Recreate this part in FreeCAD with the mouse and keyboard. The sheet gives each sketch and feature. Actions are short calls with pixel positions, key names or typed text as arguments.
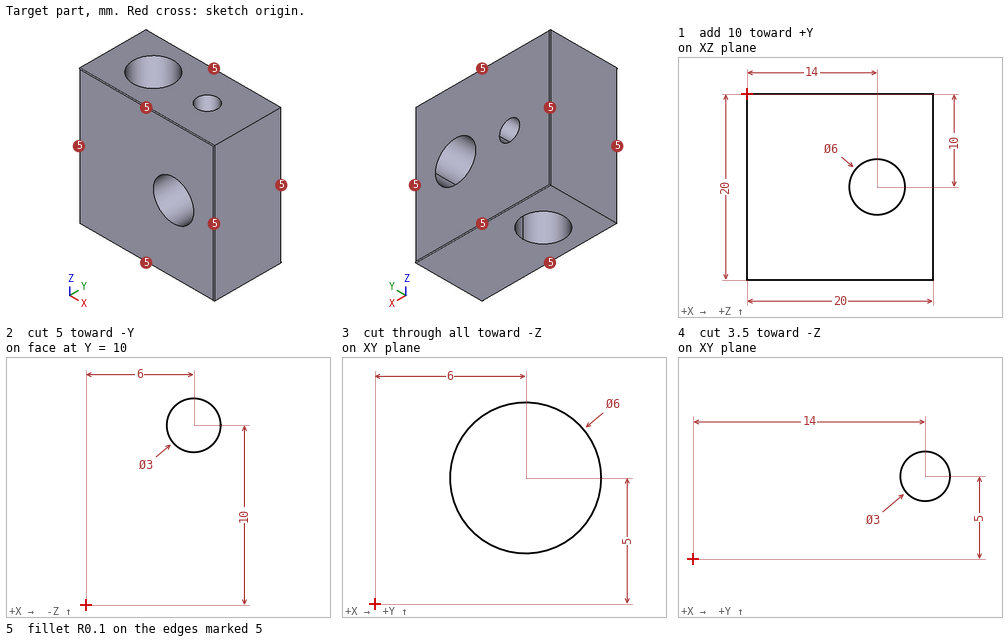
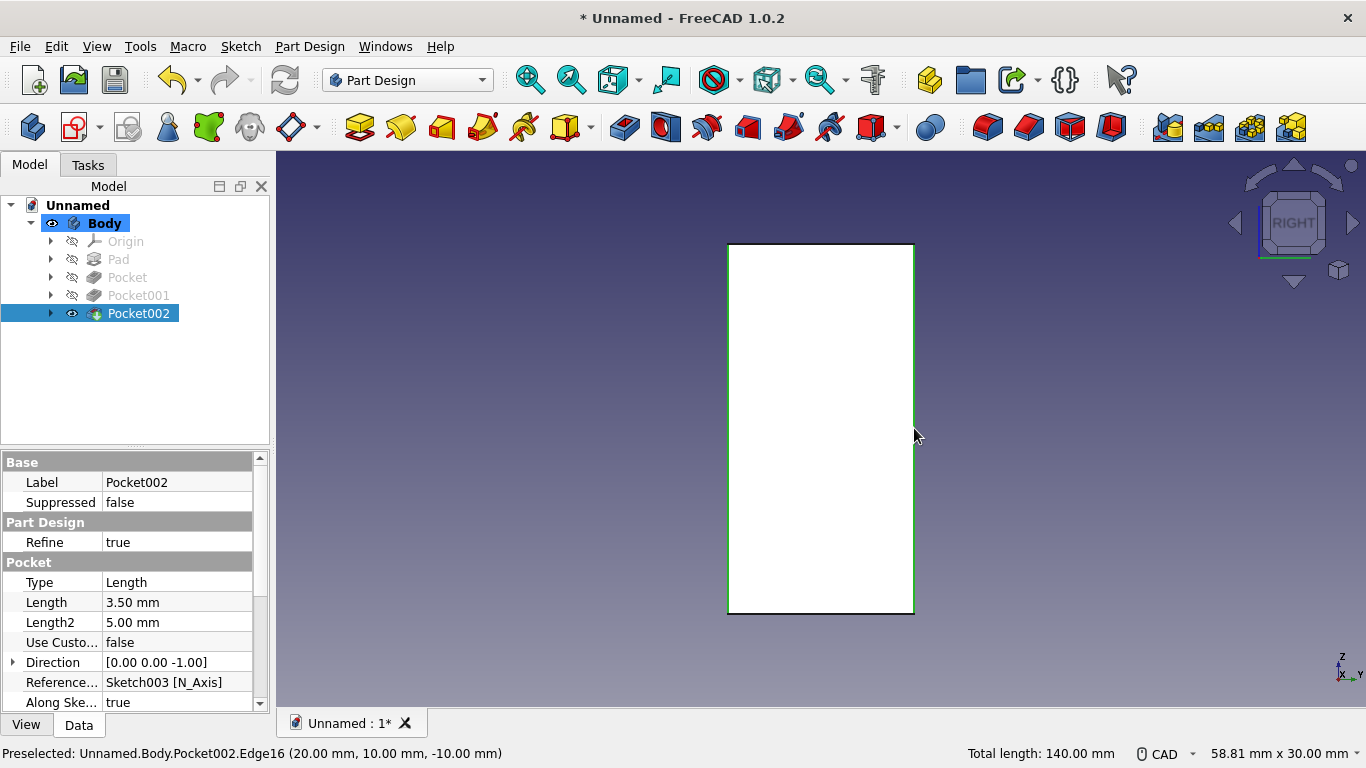
key(5)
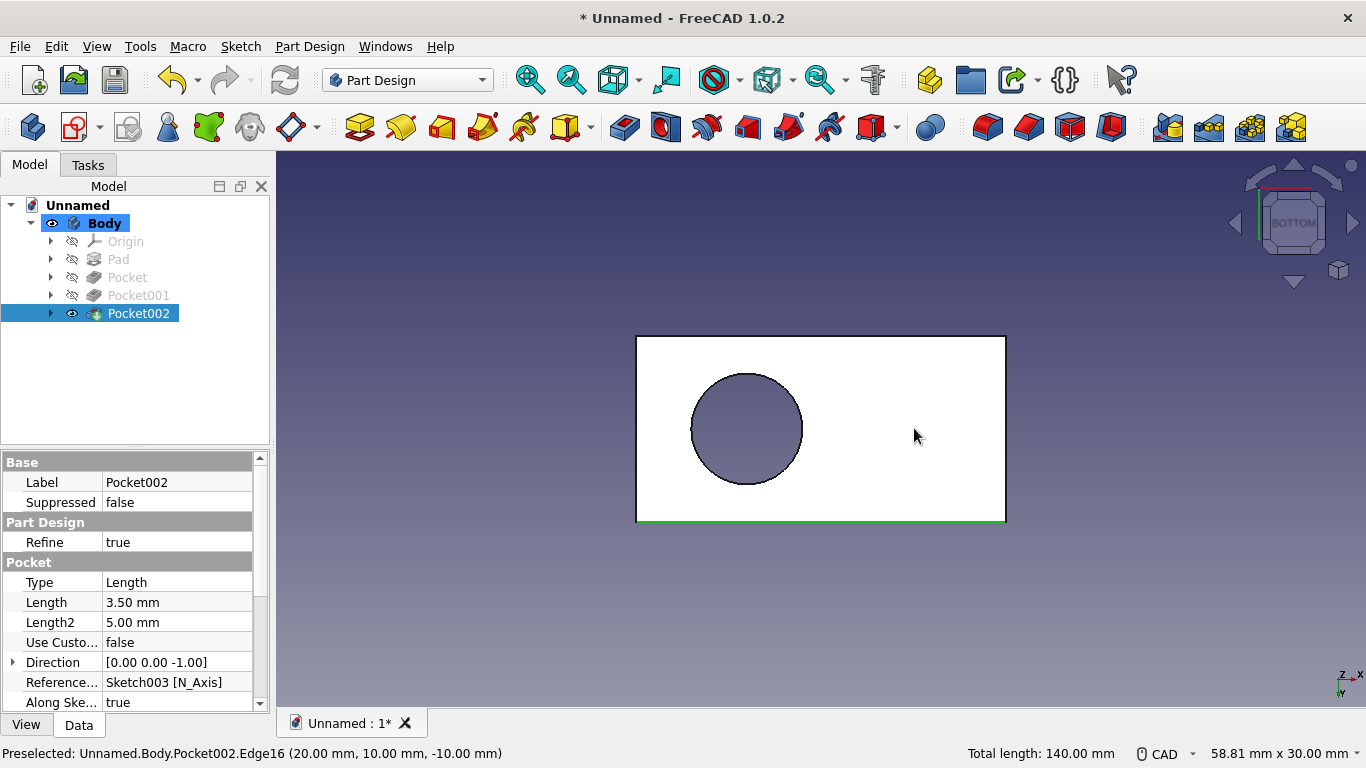
key(v)
key(f)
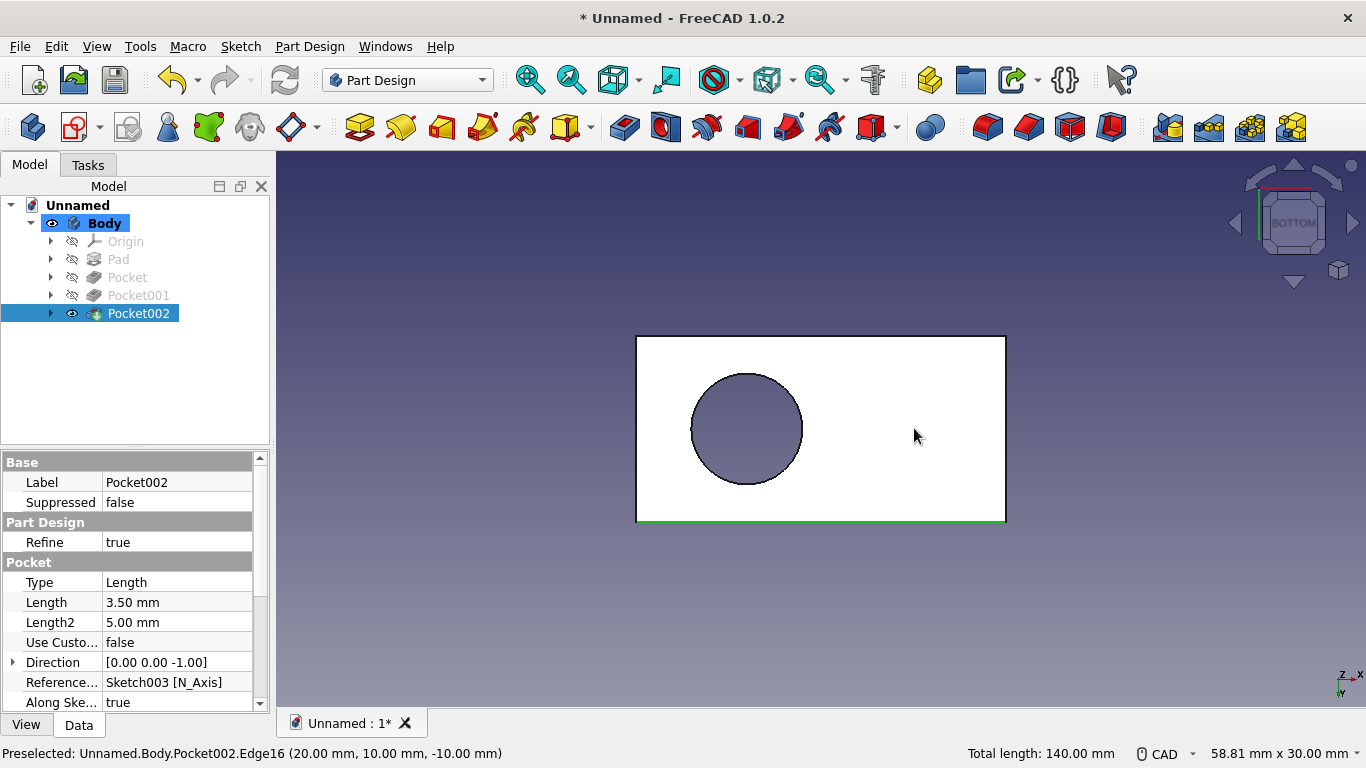
click(821, 335, ctrl)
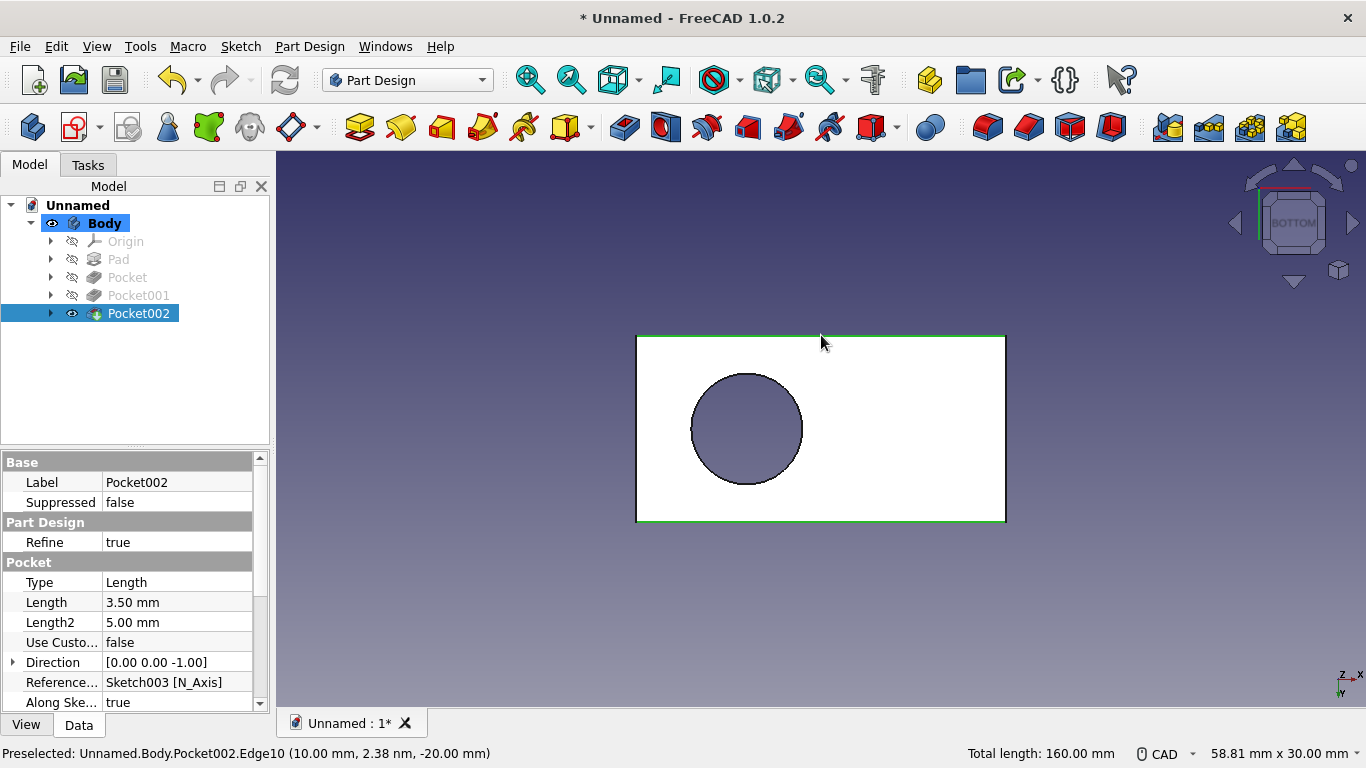
click(988, 128)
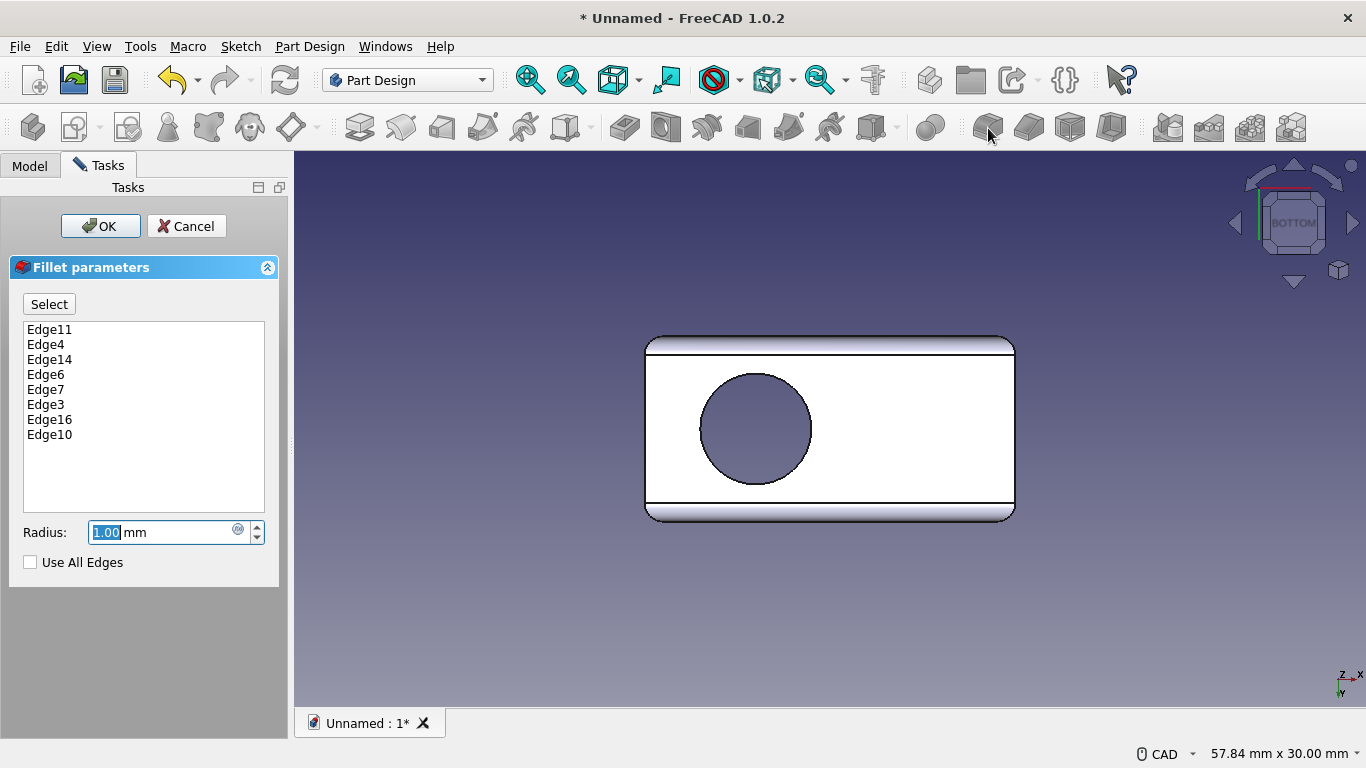
text(0.1)
key(Tab)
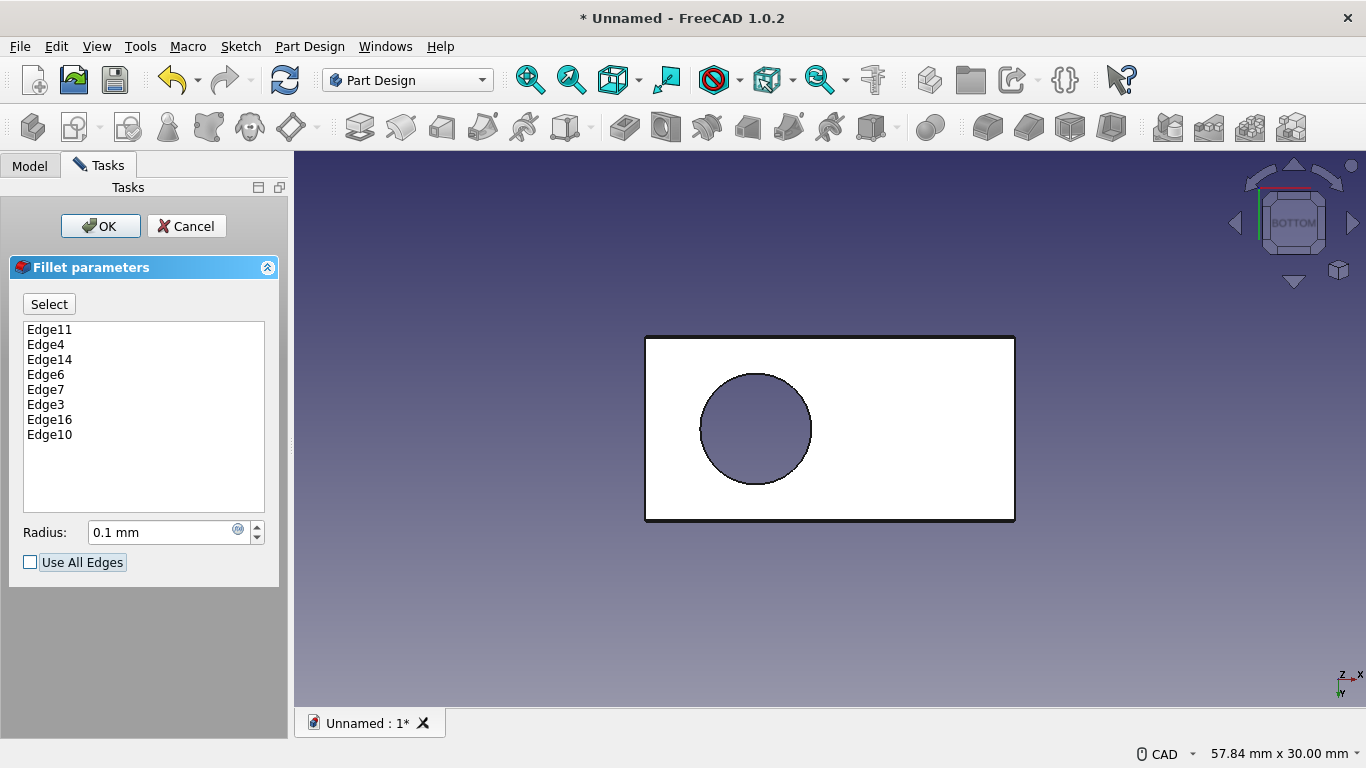
click(101, 226)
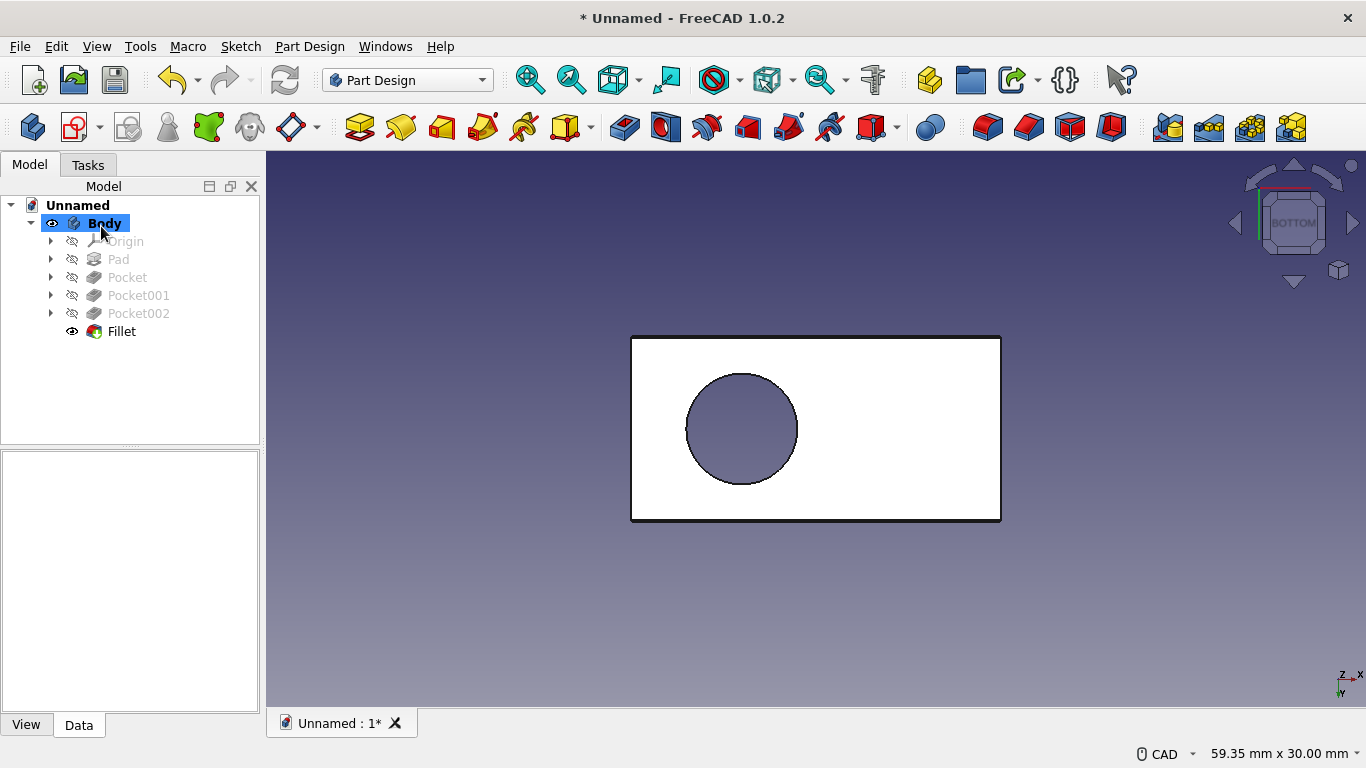
key(0)